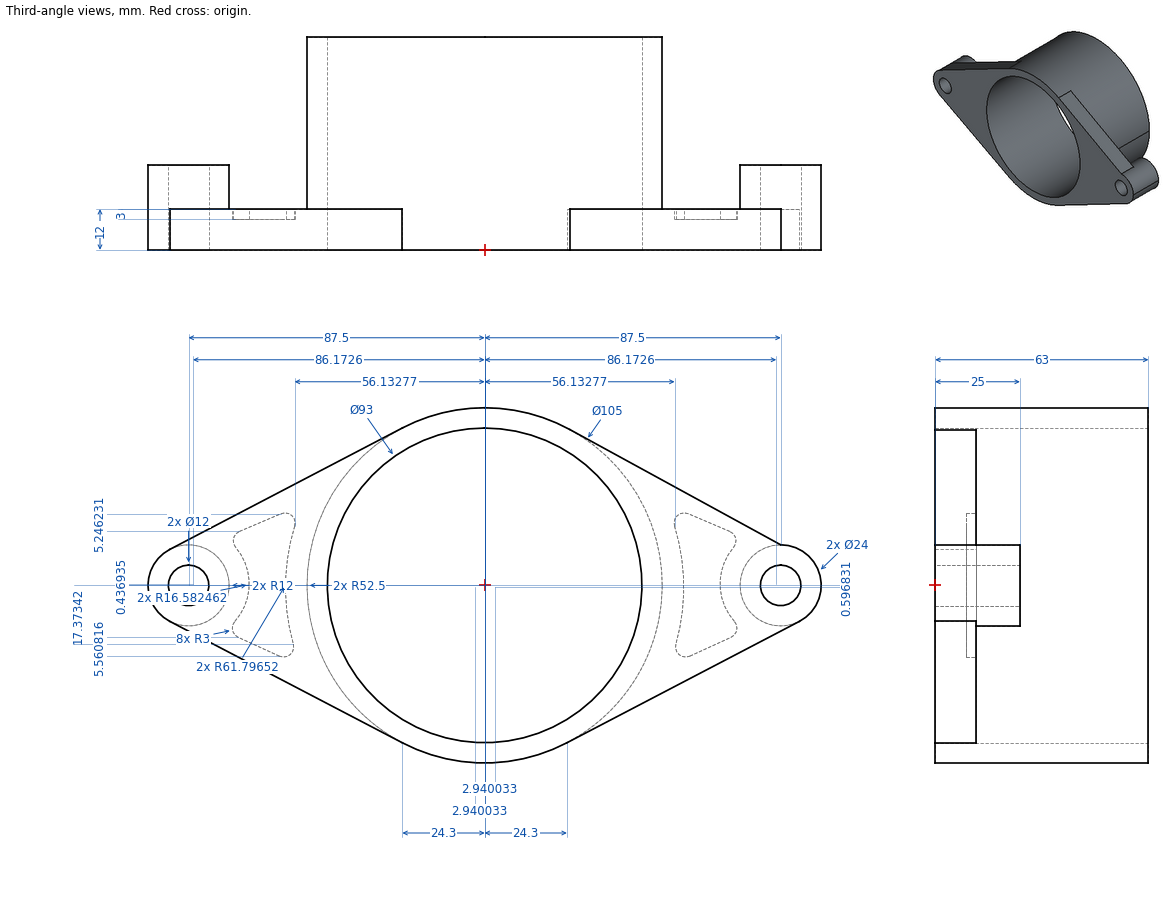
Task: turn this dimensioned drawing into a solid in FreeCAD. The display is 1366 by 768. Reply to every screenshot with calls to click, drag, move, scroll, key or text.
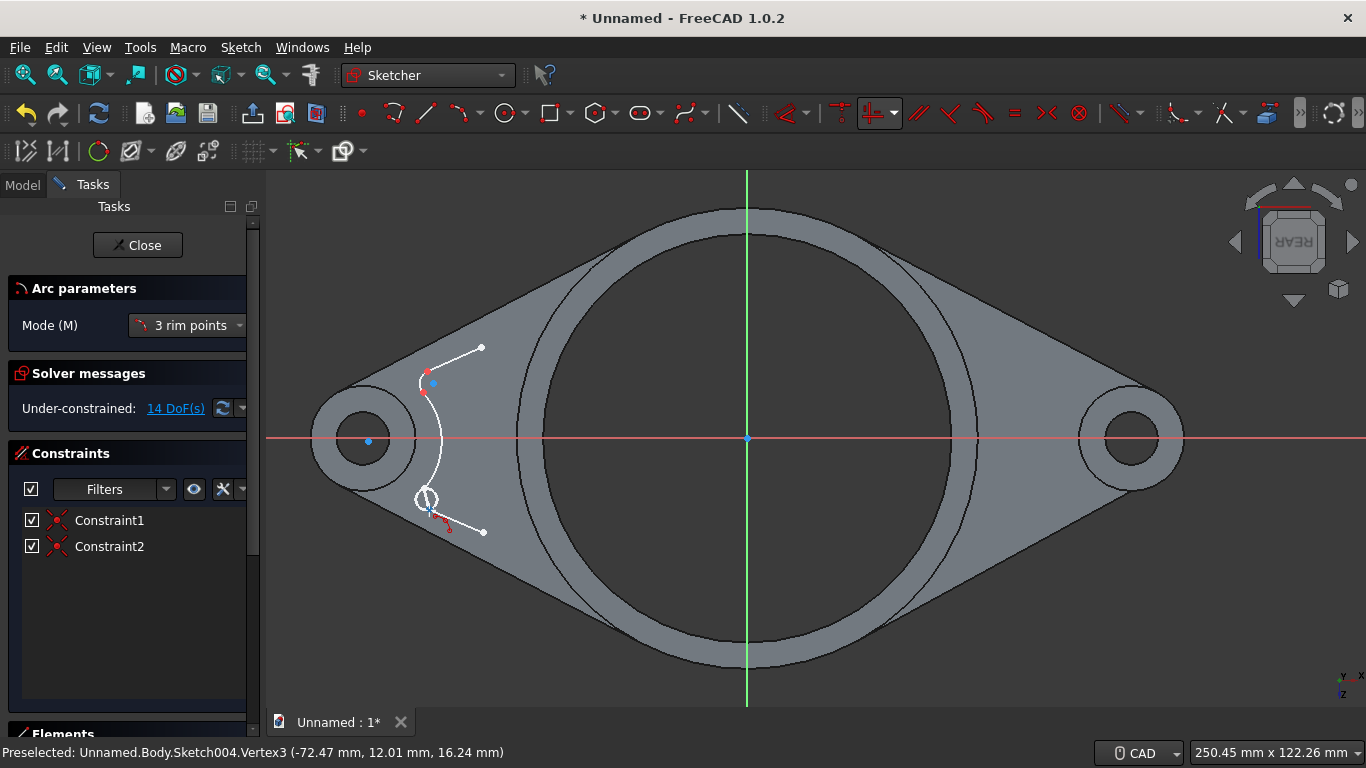
scroll(421, 499, up, 6)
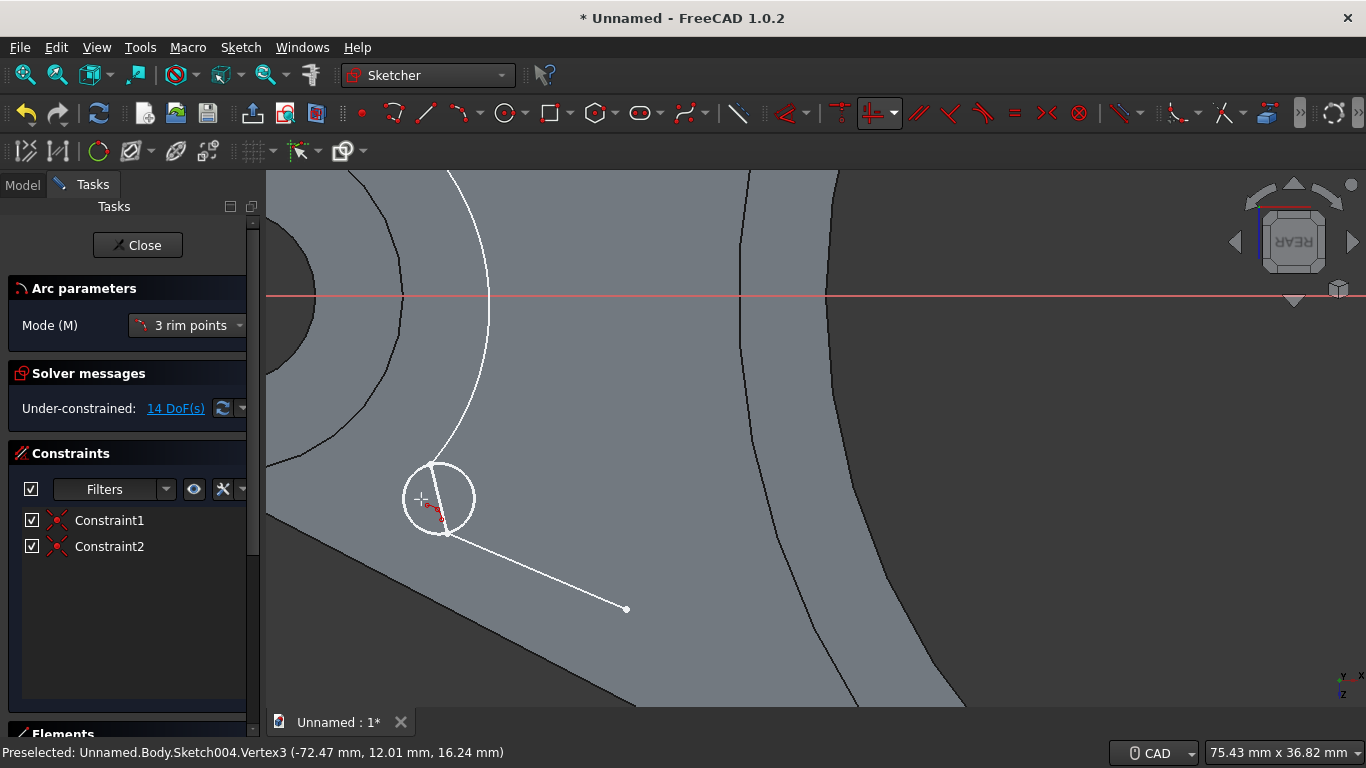
click(422, 498)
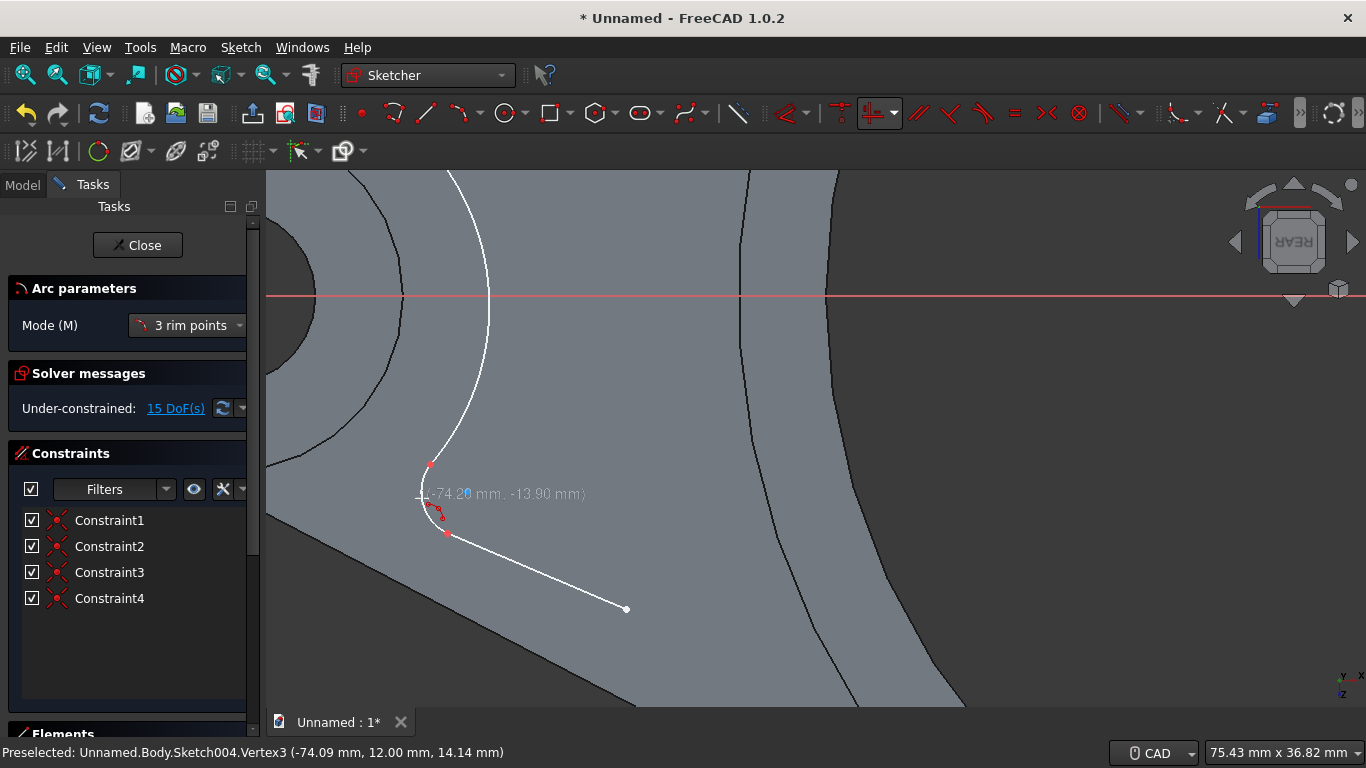
click(627, 609)
click(685, 552)
click(673, 598)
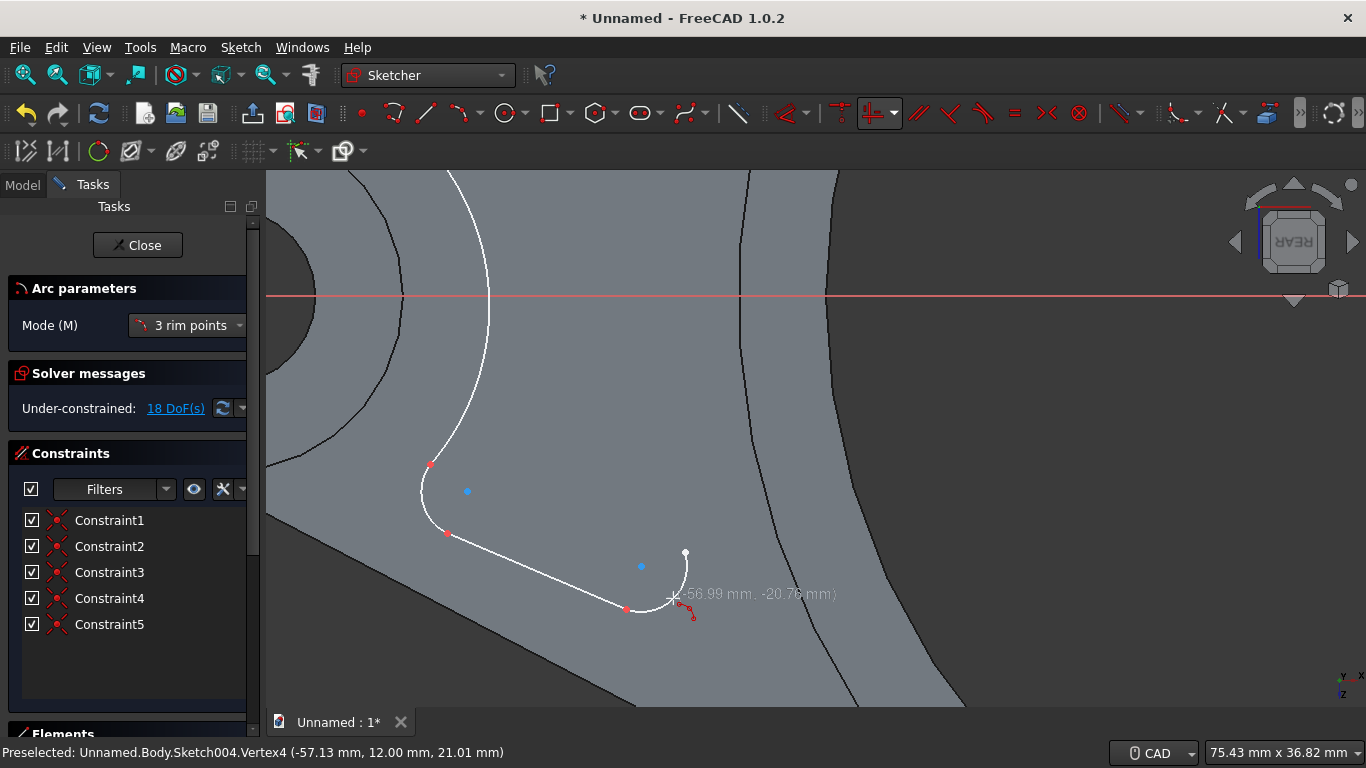
click(685, 553)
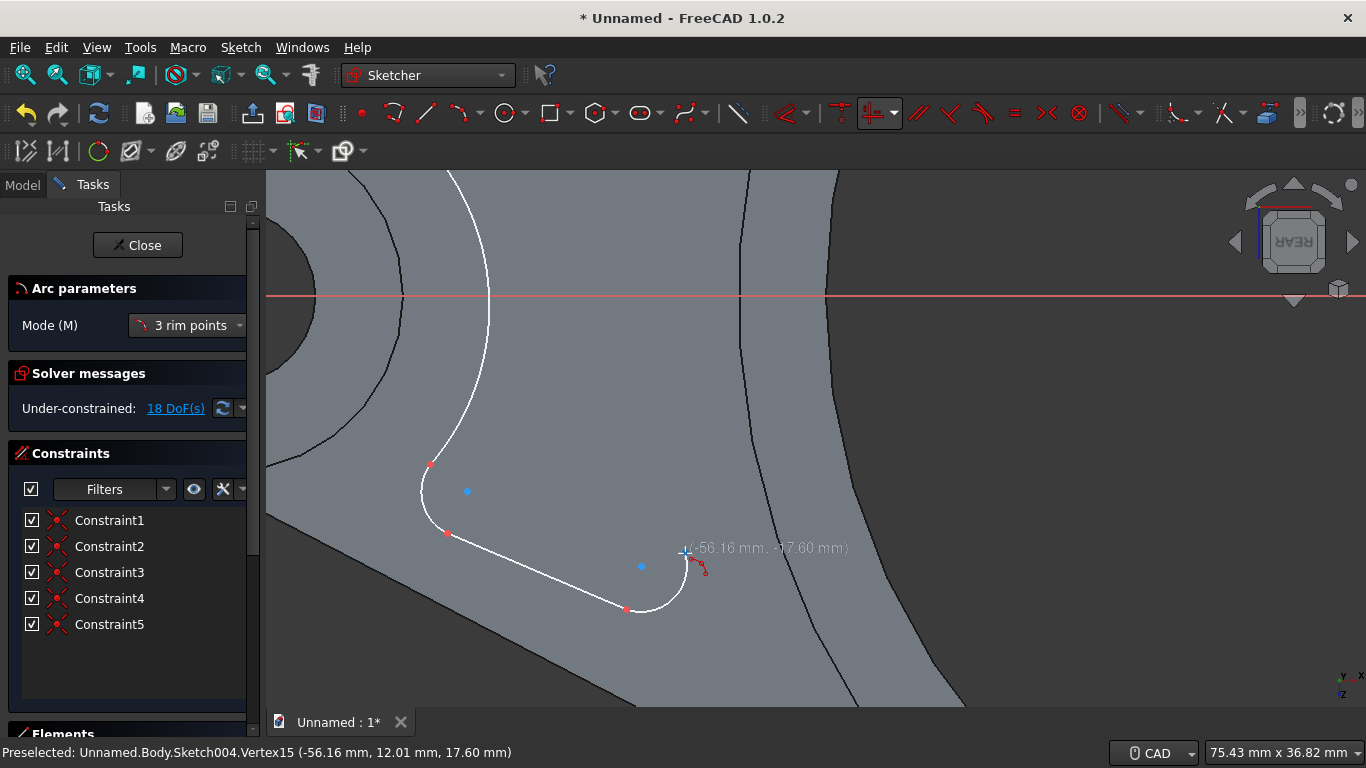
scroll(421, 499, down, 6)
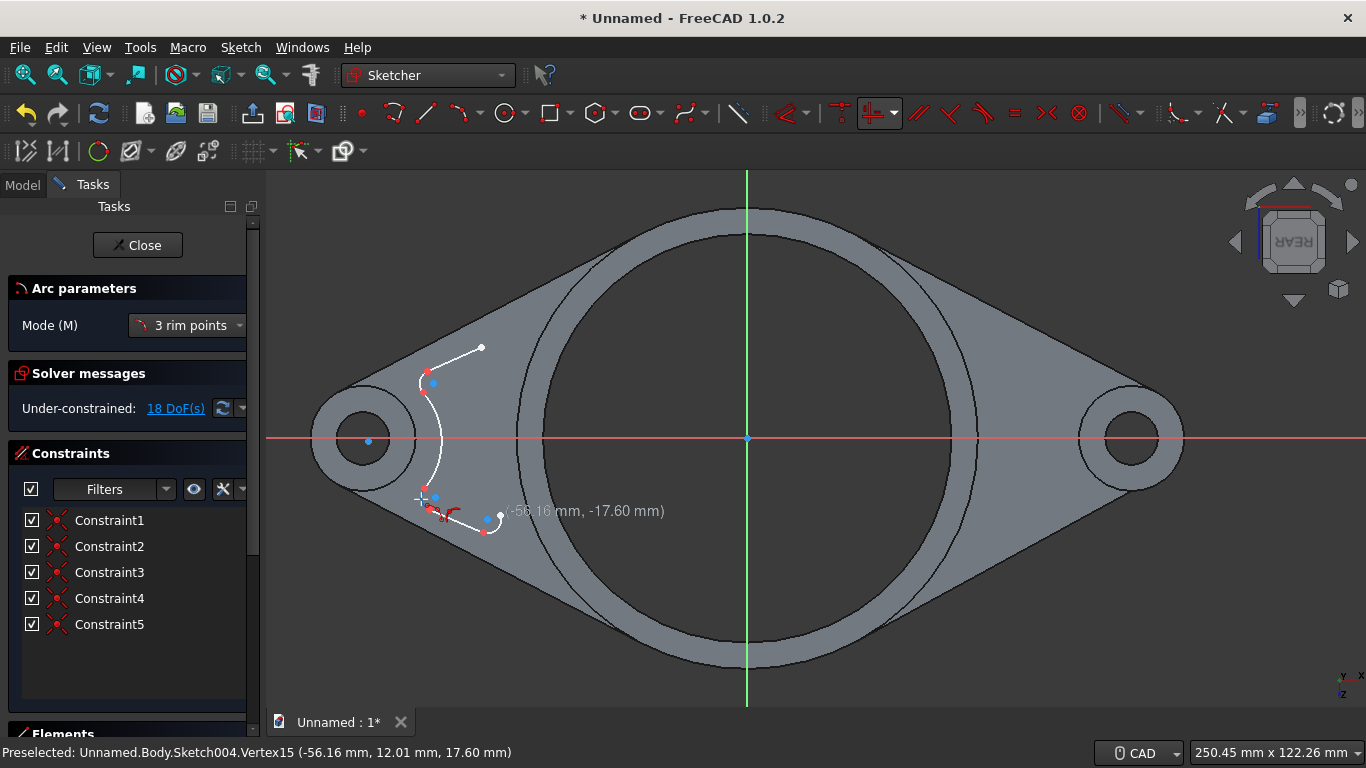
click(499, 362)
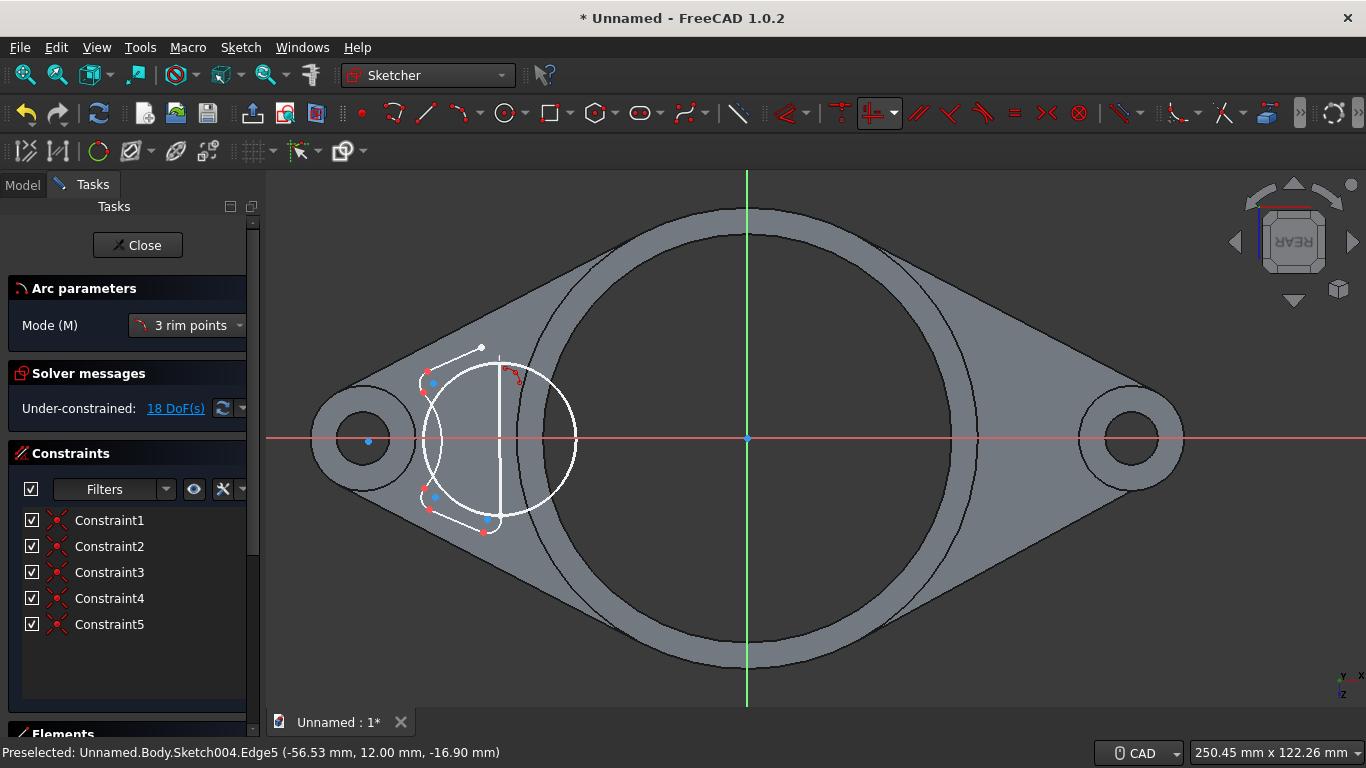
scroll(489, 423, up, 3)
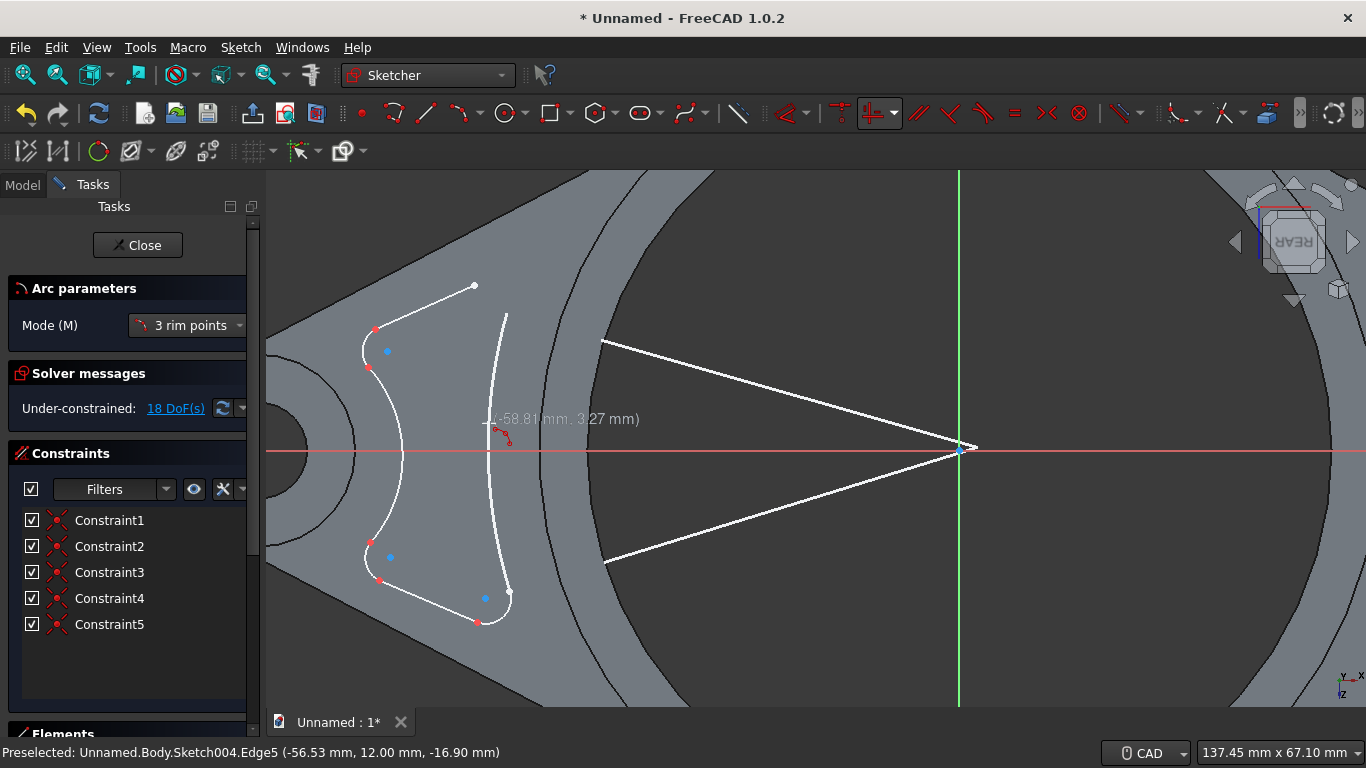
click(489, 423)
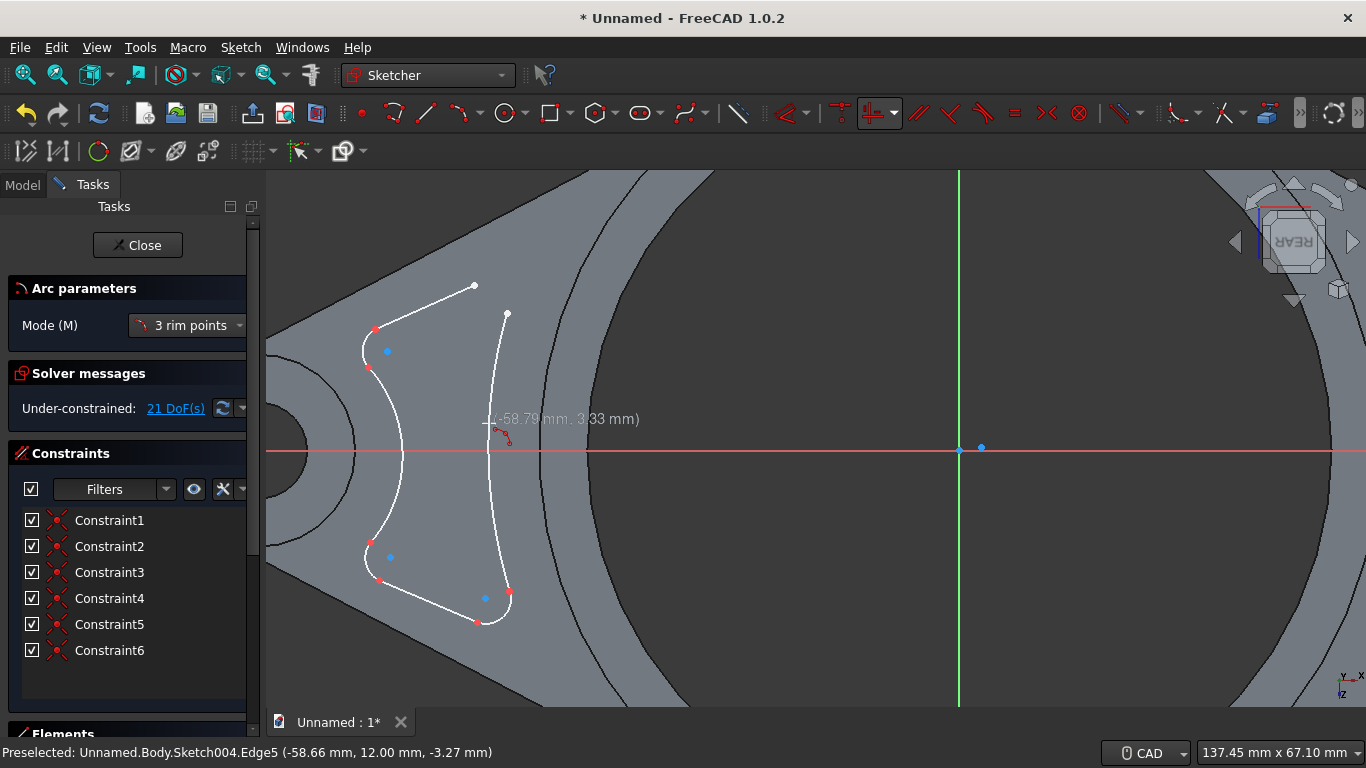
click(507, 313)
click(474, 285)
click(500, 287)